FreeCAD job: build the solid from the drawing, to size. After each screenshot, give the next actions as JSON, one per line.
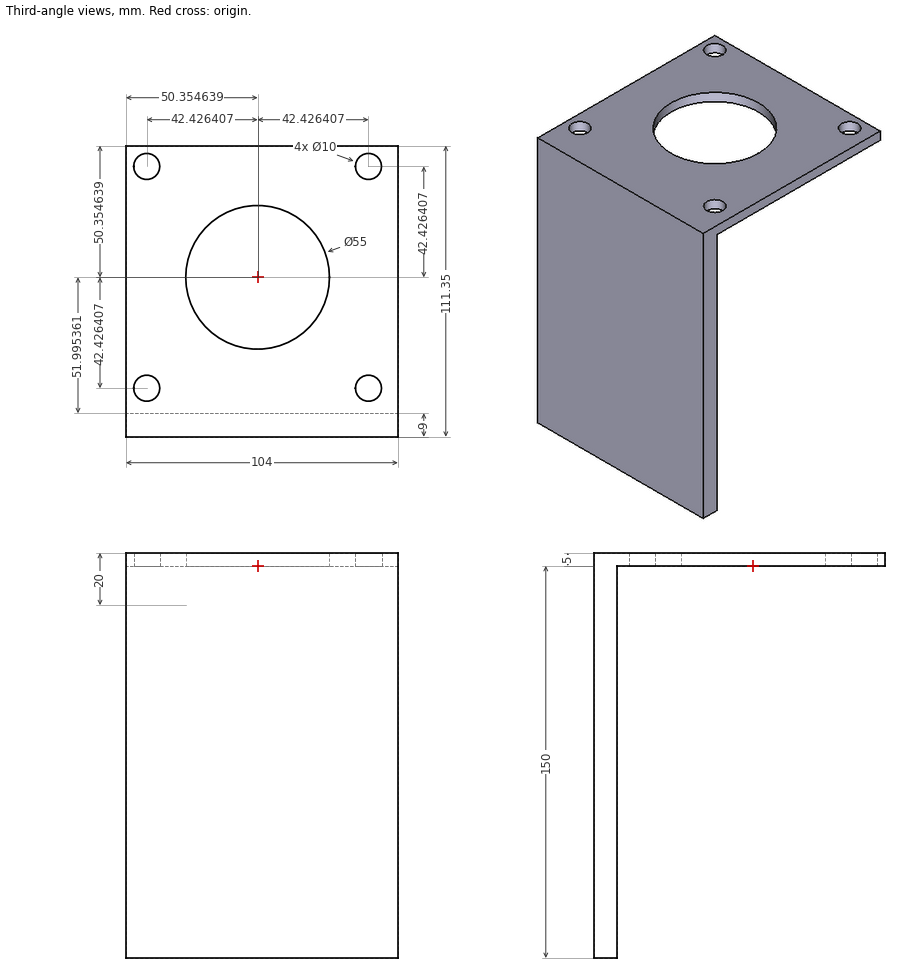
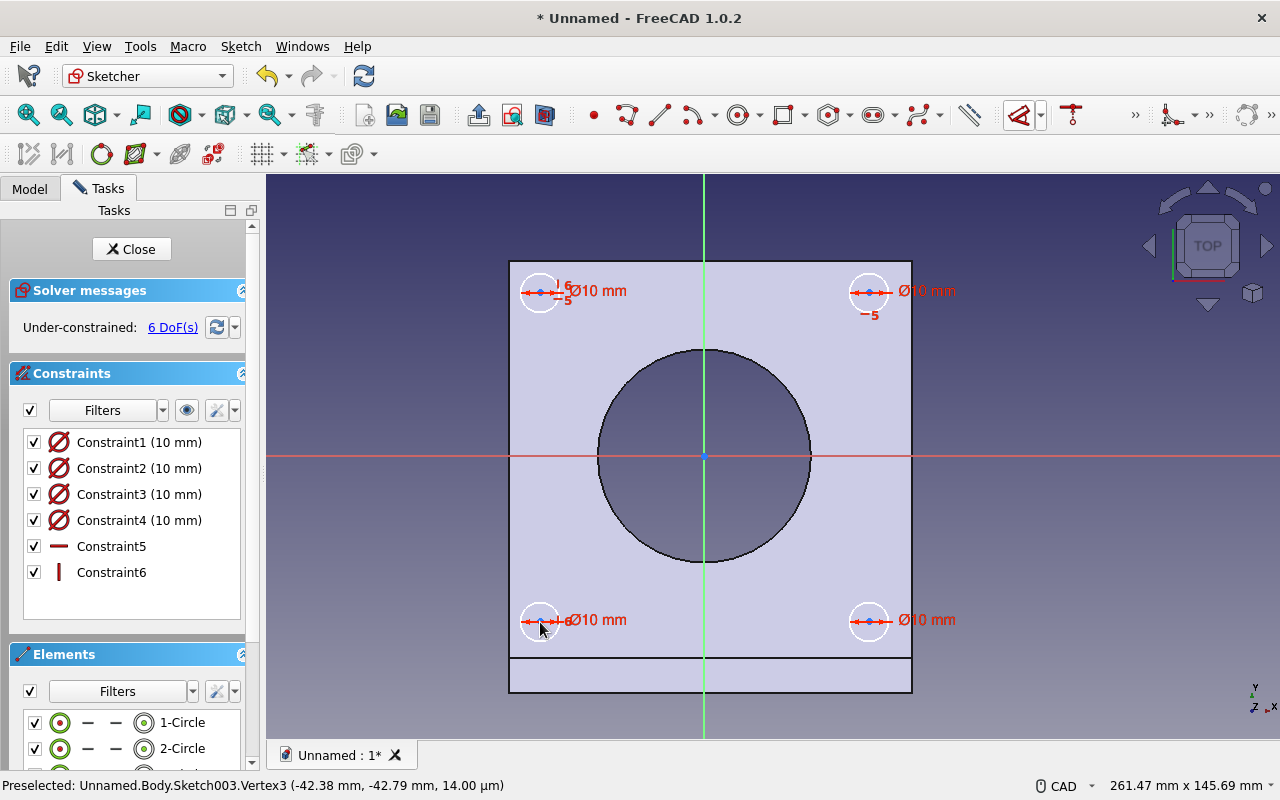
{"action": "left_click", "coordinate": [869, 293]}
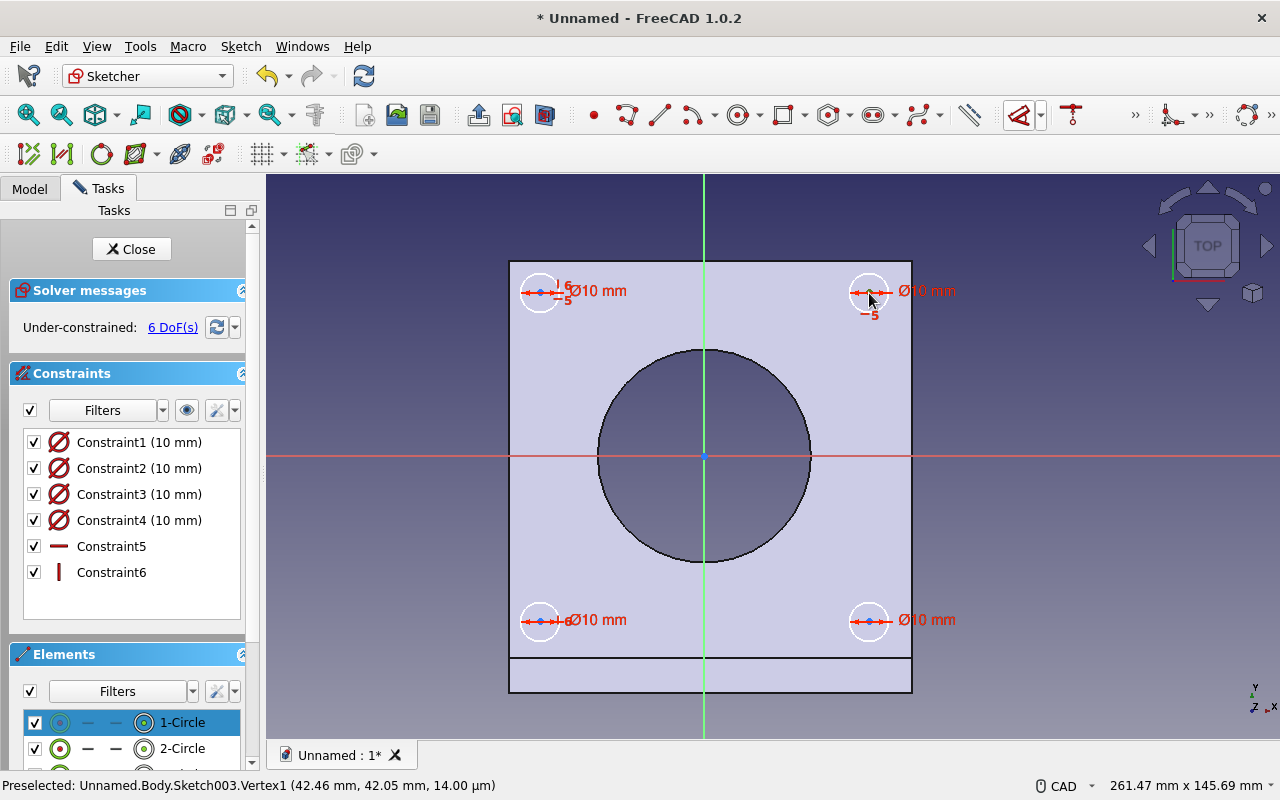
{"action": "left_click", "coordinate": [869, 622]}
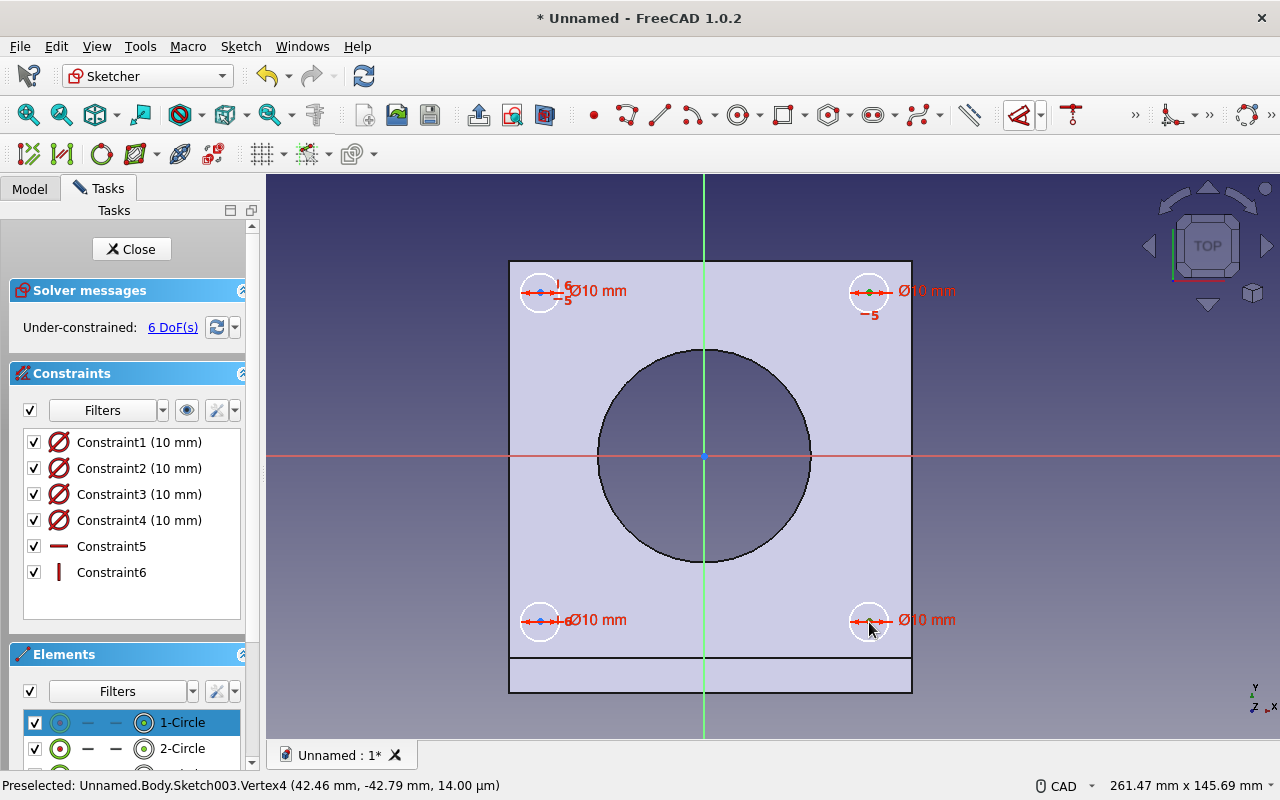
{"action": "key", "text": "v"}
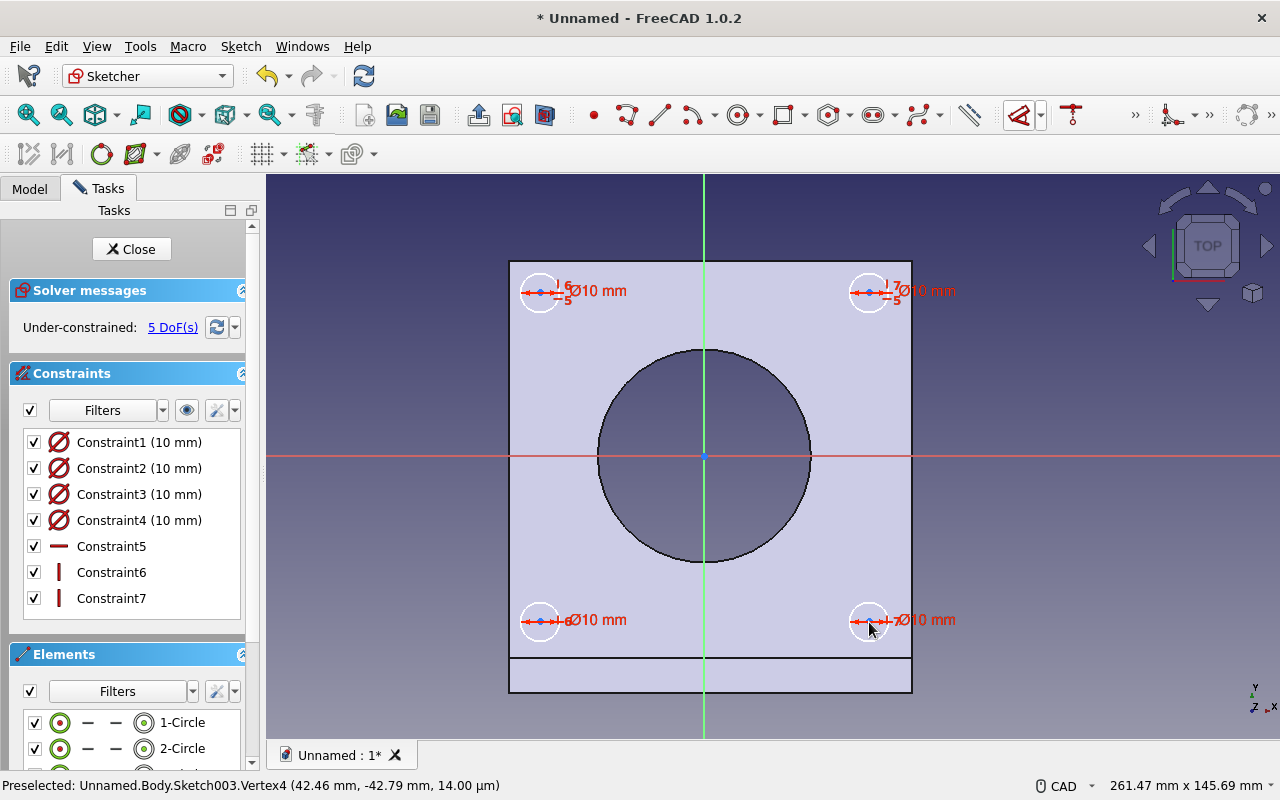
{"action": "left_click", "coordinate": [540, 622]}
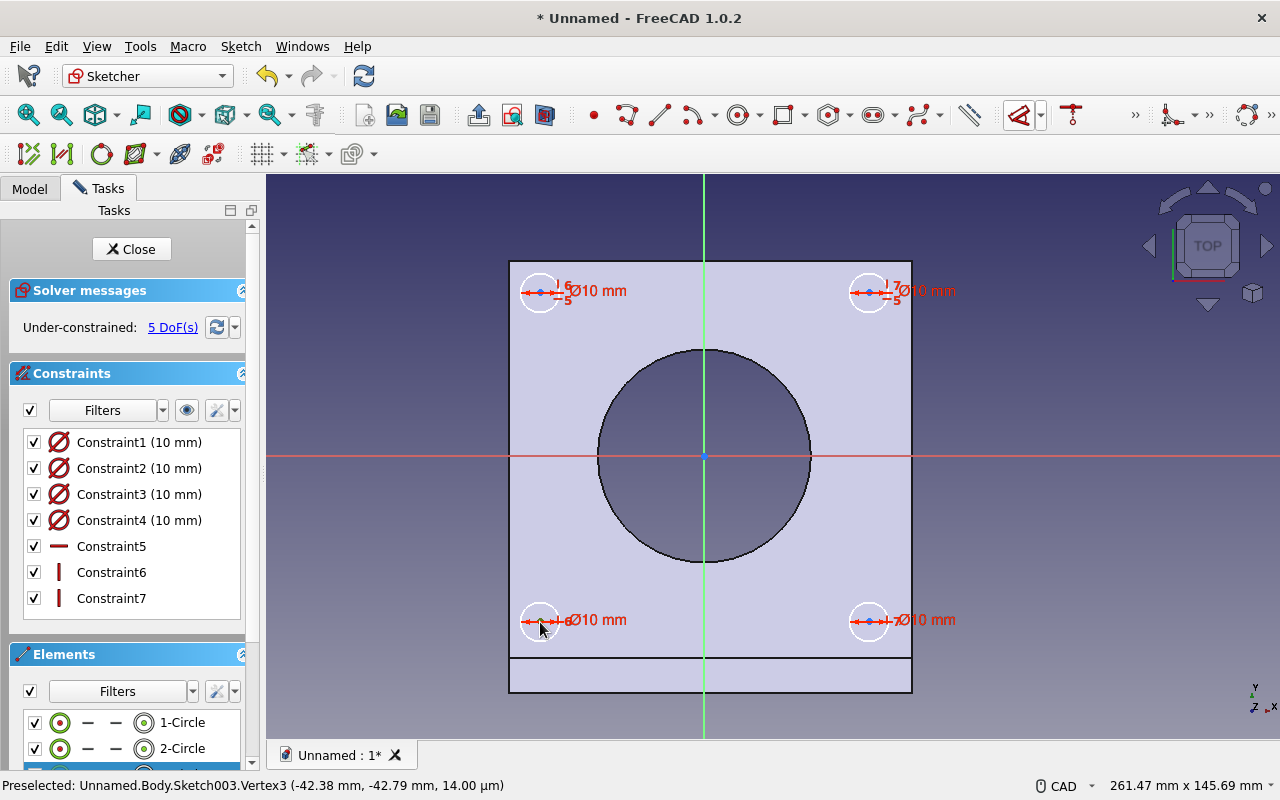
{"action": "left_click", "coordinate": [869, 622]}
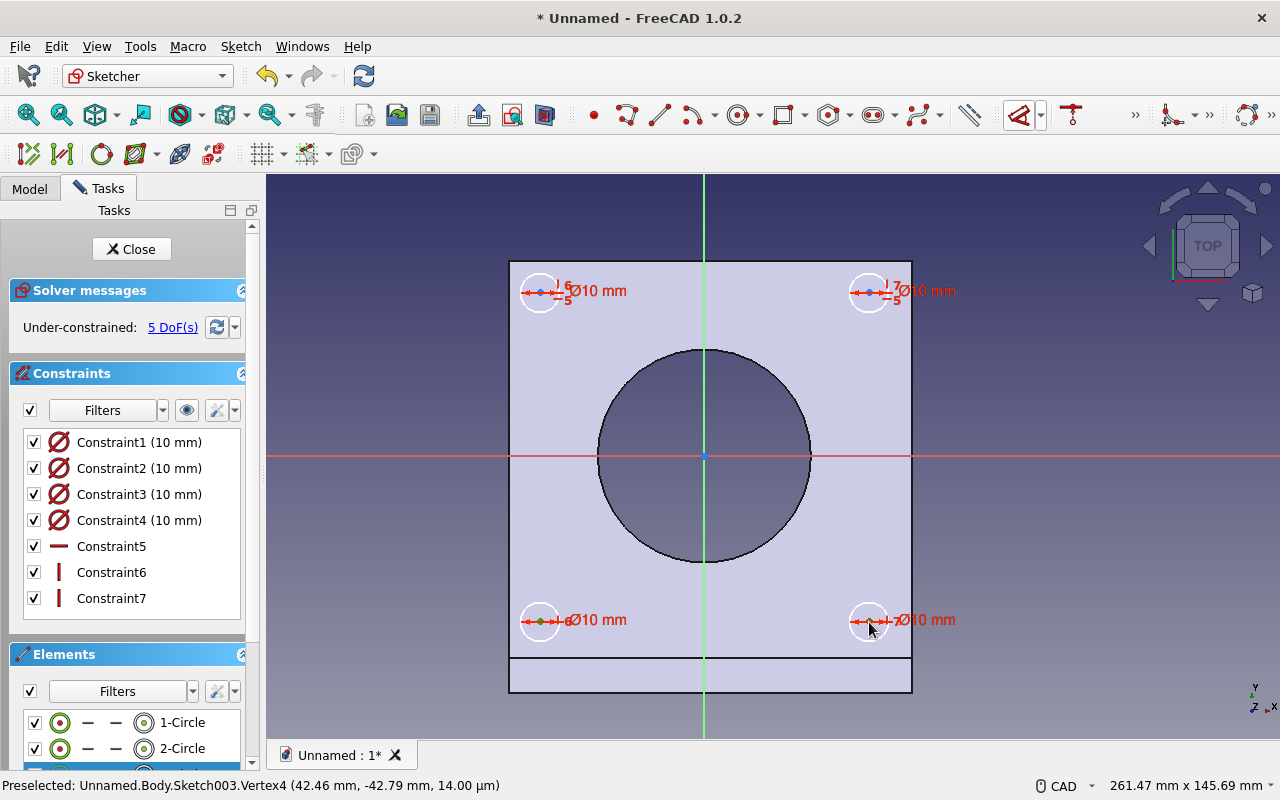
{"action": "key", "text": "h"}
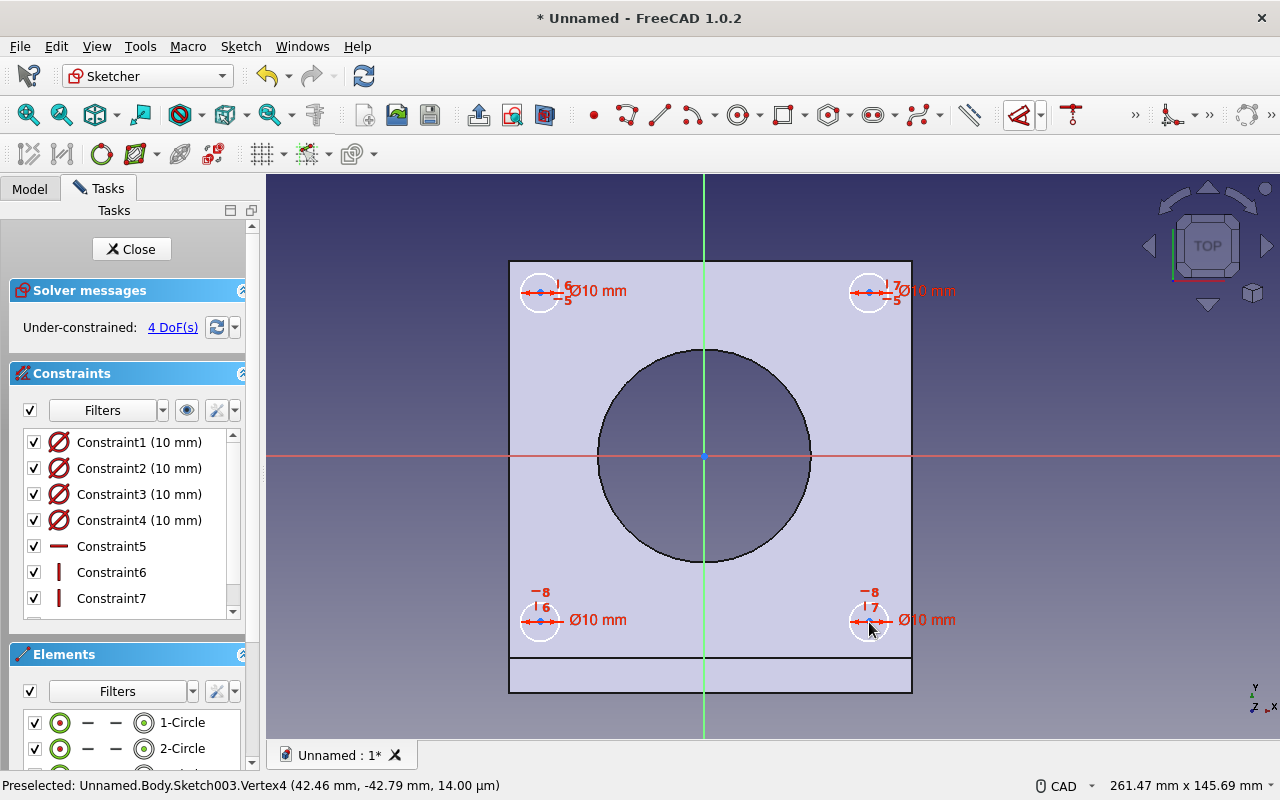
{"action": "left_click", "coordinate": [869, 293]}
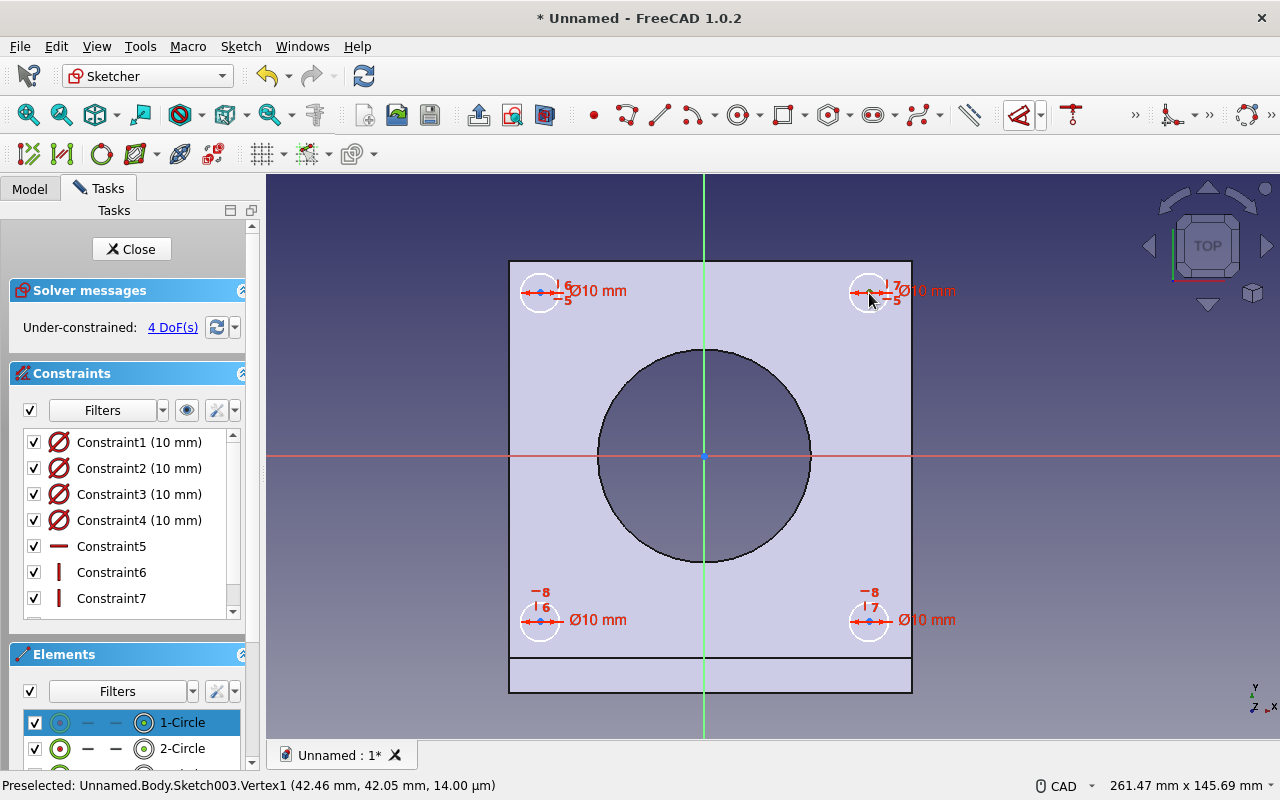
{"action": "left_click", "coordinate": [1040, 116]}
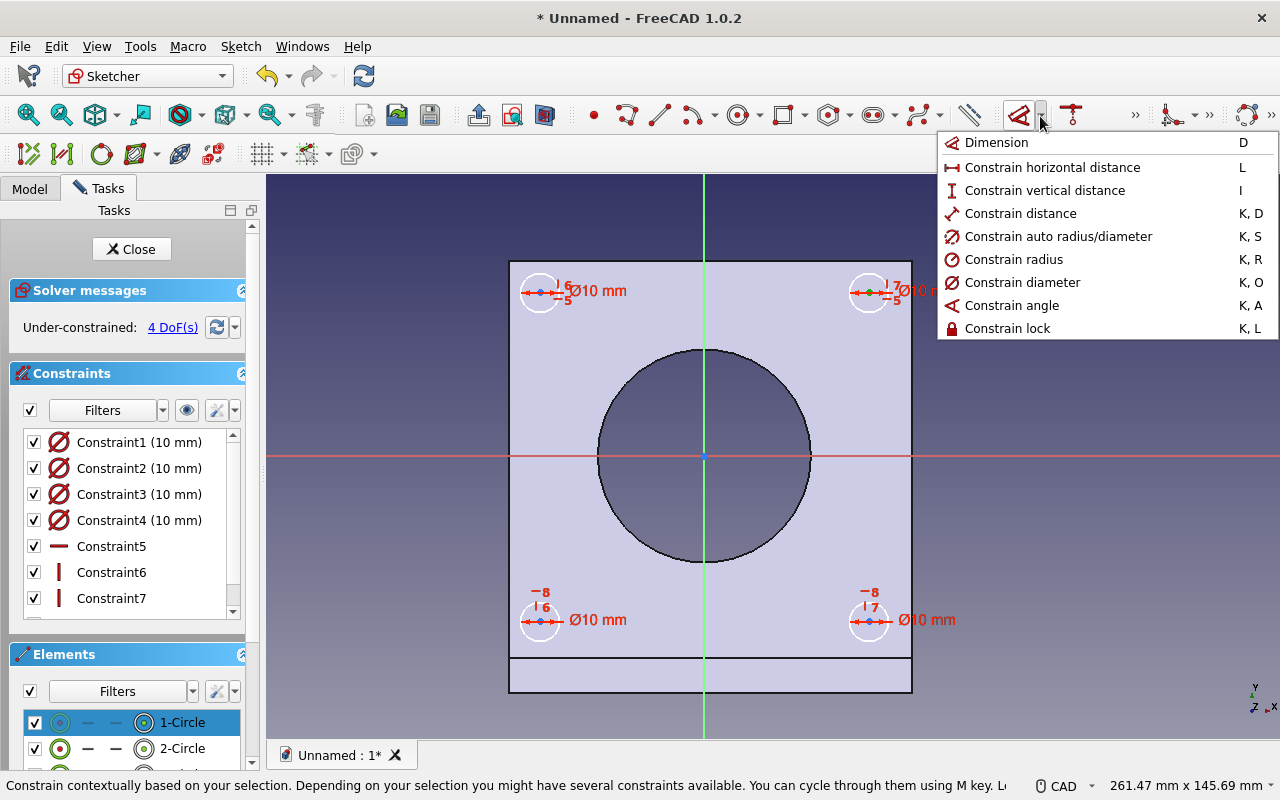
{"action": "left_click", "coordinate": [1108, 168]}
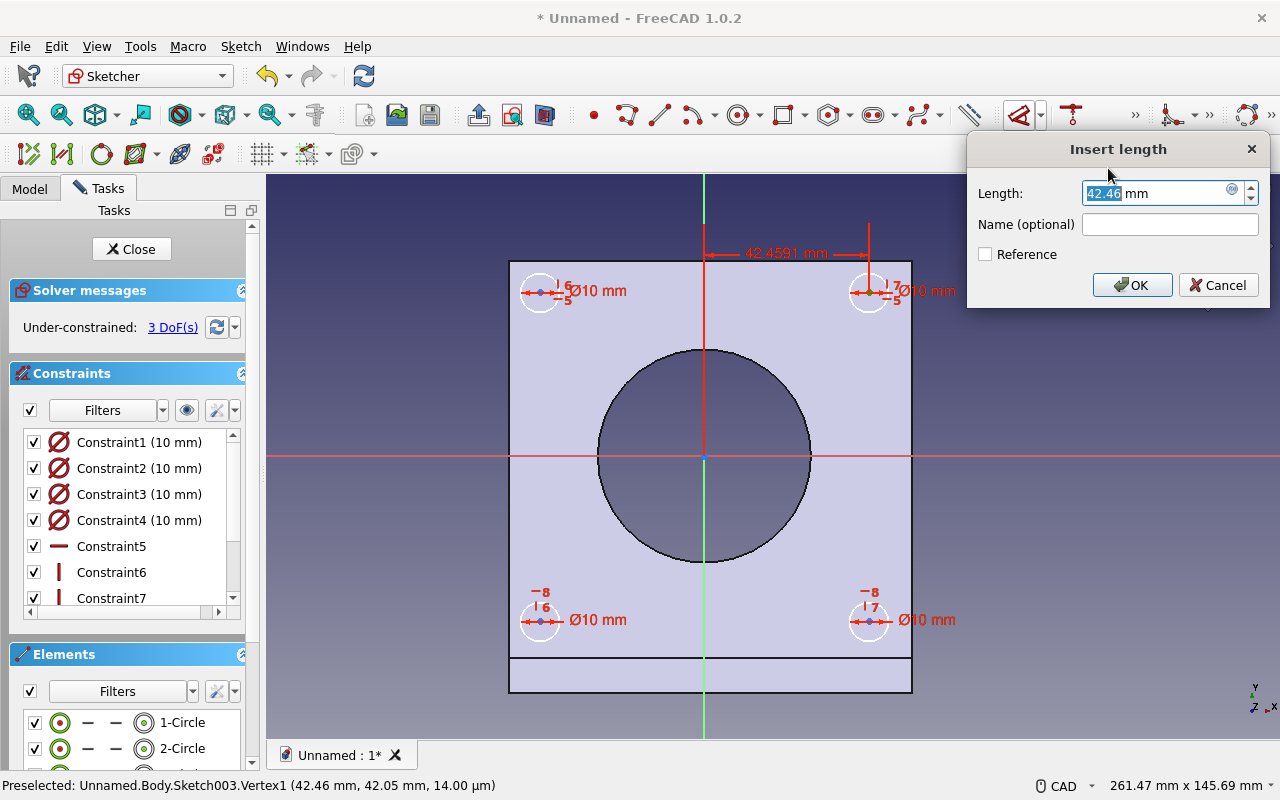
{"action": "type", "text": "42.426407"}
{"action": "key", "text": "Return"}